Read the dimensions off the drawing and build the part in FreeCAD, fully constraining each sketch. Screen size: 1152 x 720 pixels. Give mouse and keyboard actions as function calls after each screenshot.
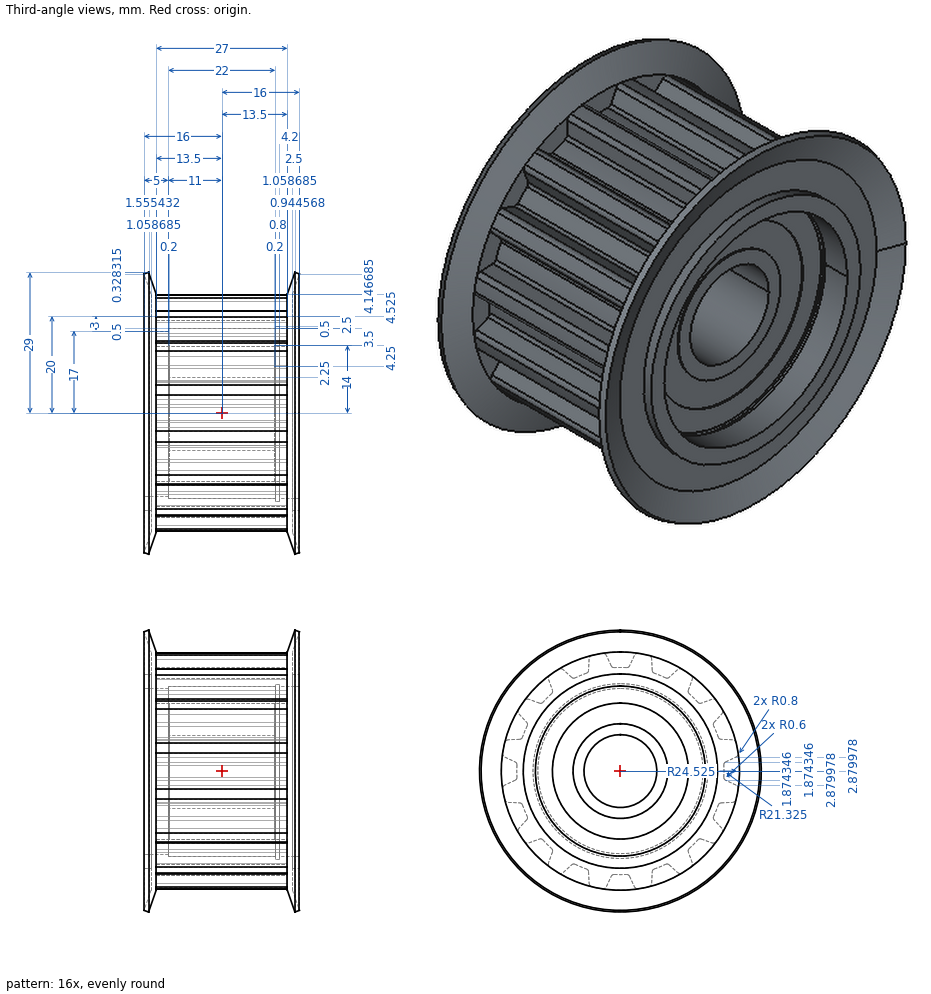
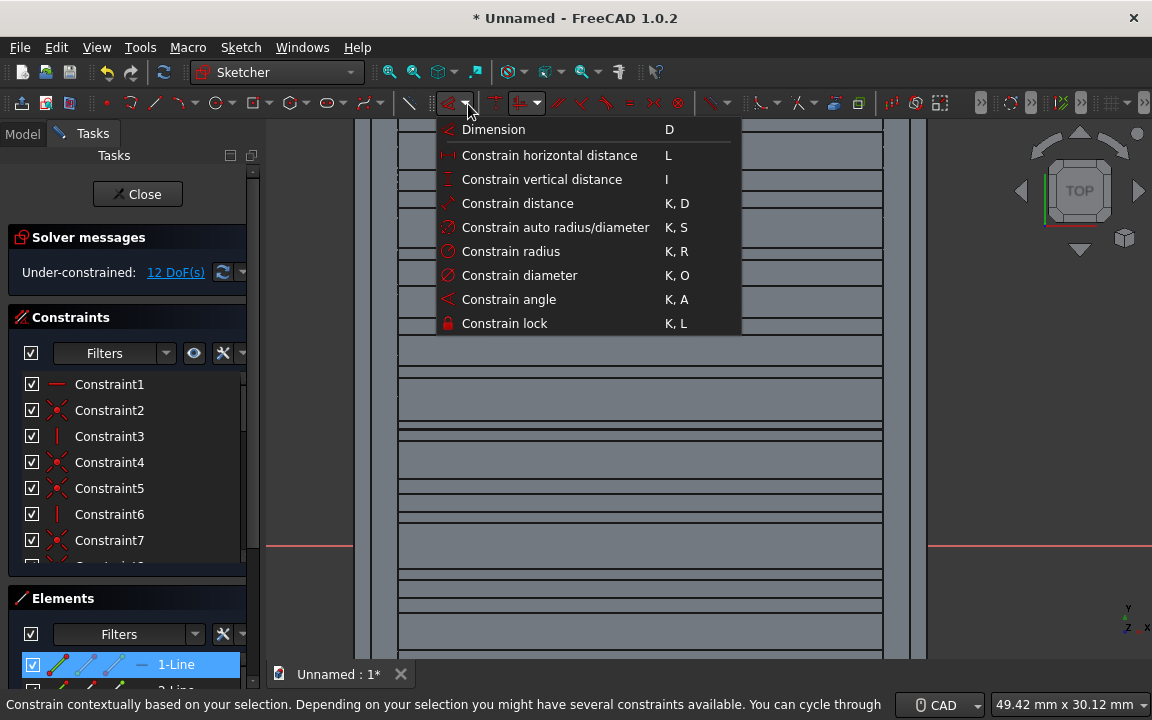
click(589, 155)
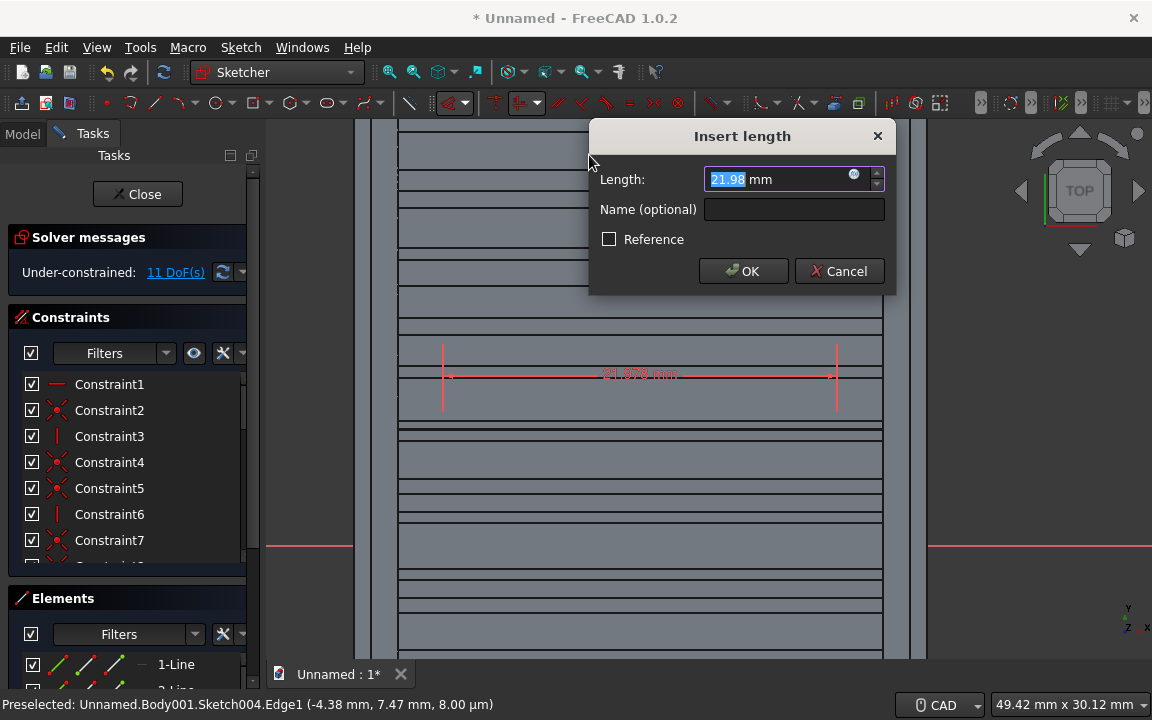
text(22)
key(Return)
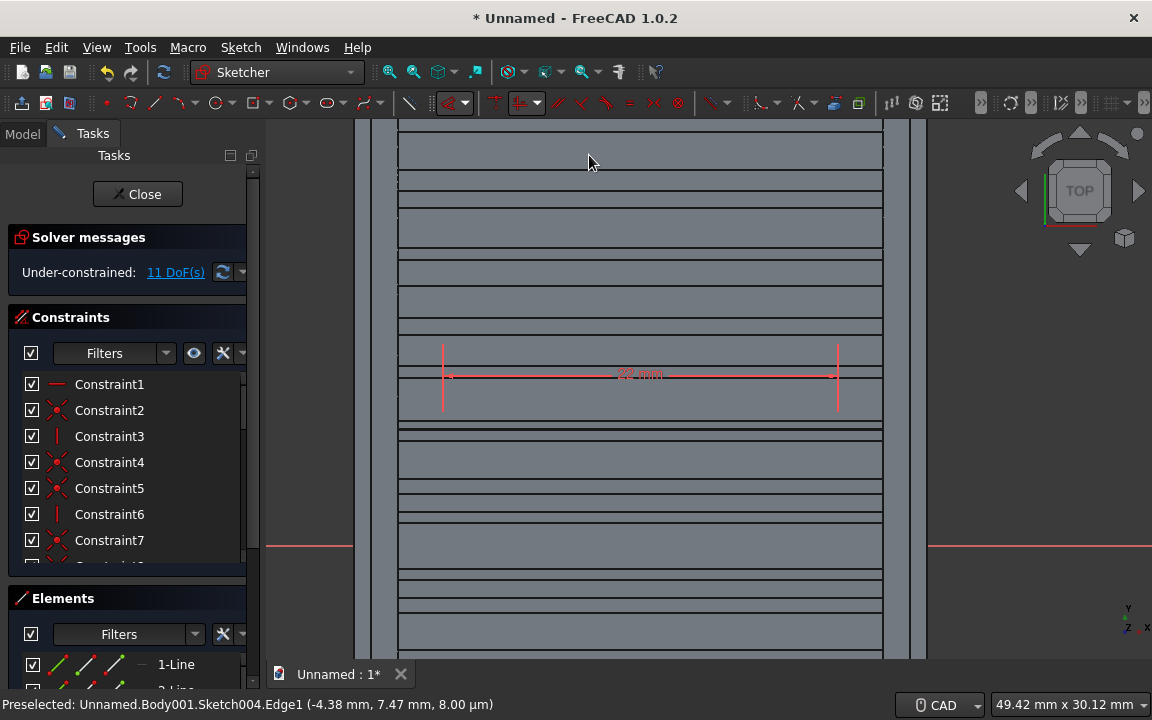
click(719, 233)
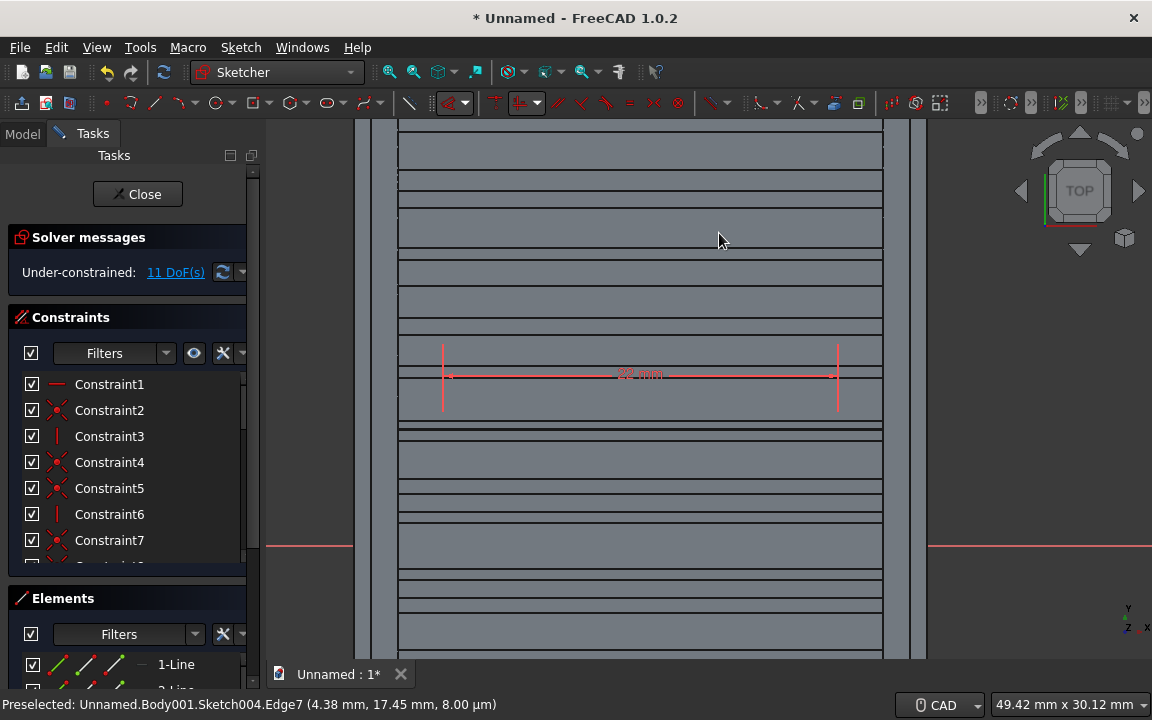
click(468, 104)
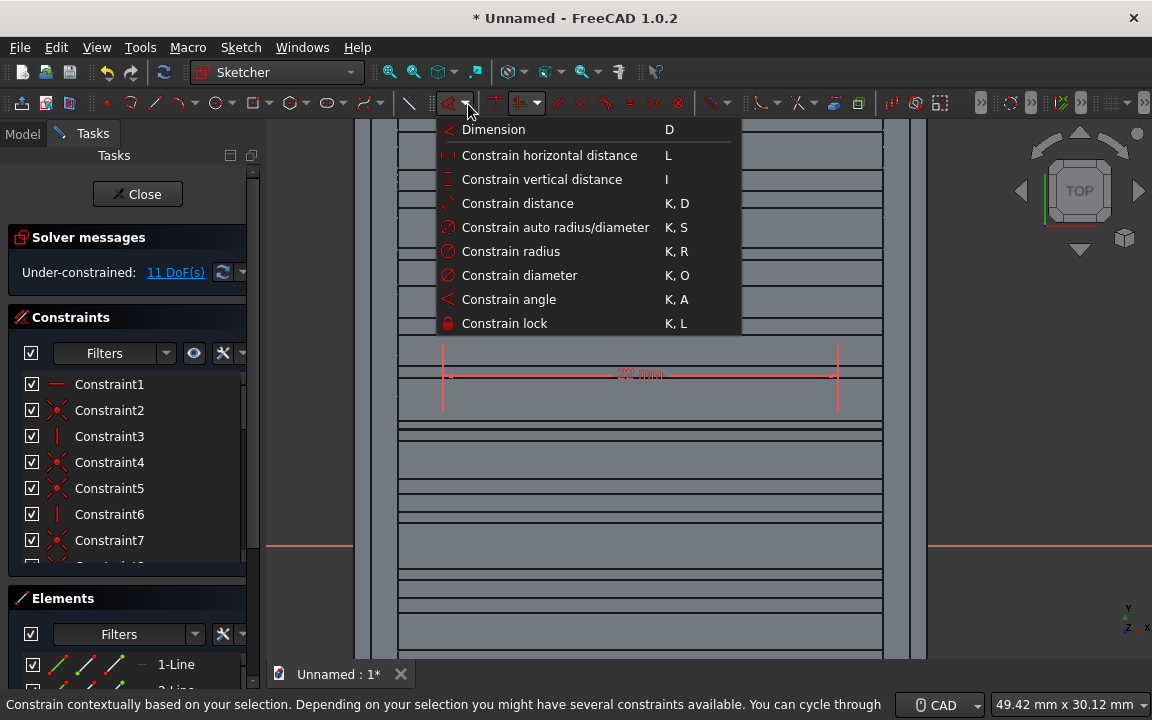
click(589, 155)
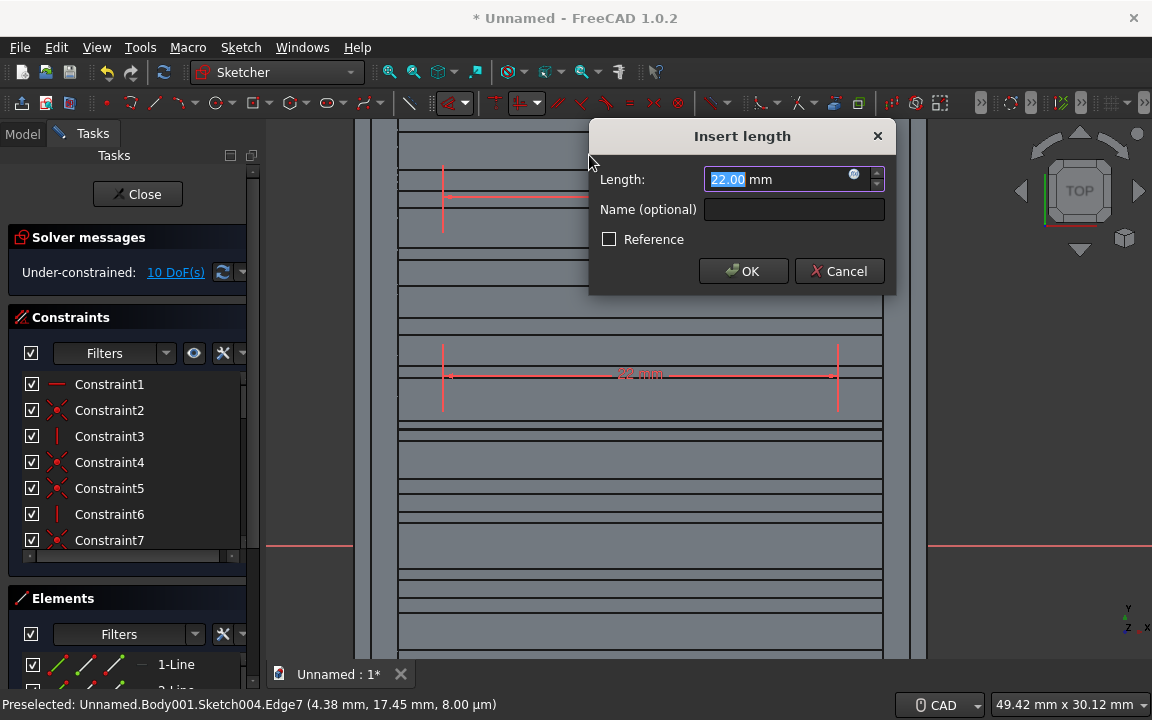
text(22)
key(Return)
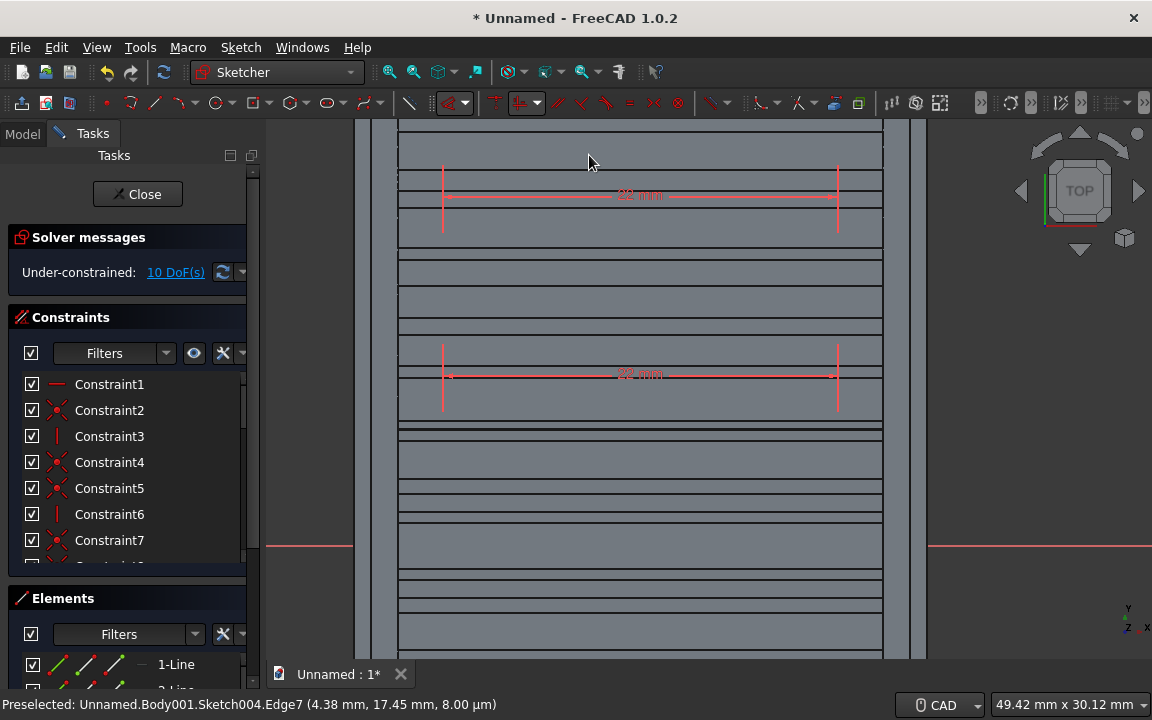
scroll(836, 372, up, 13)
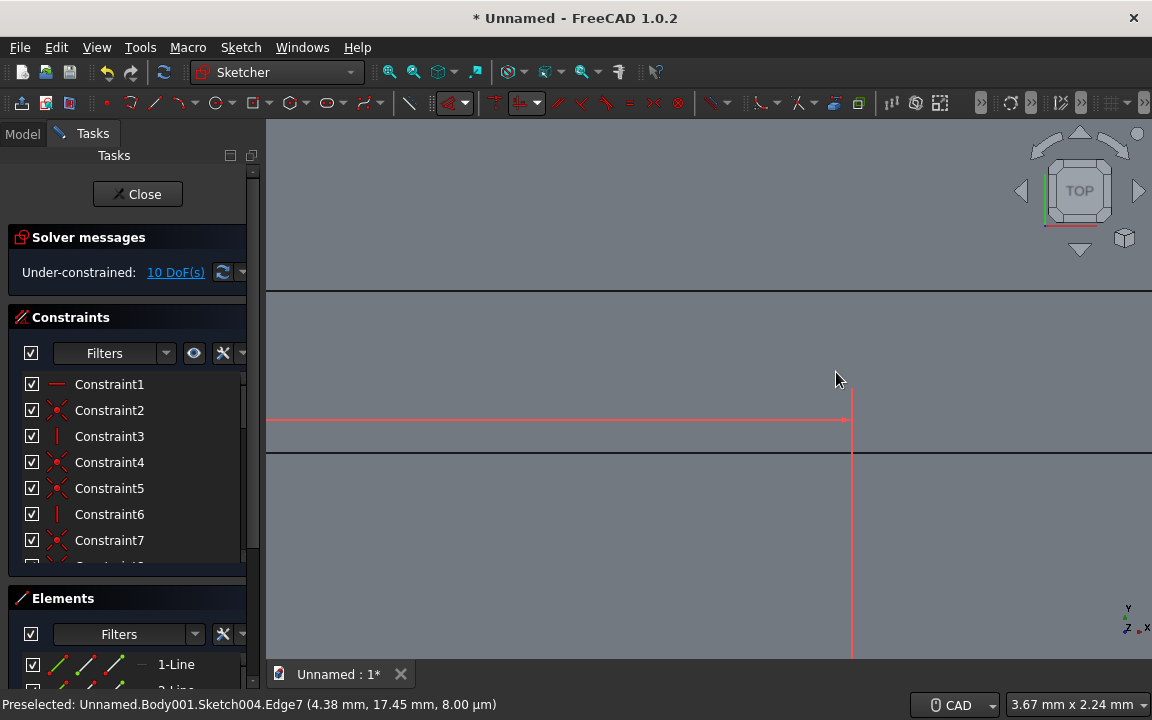
click(827, 366)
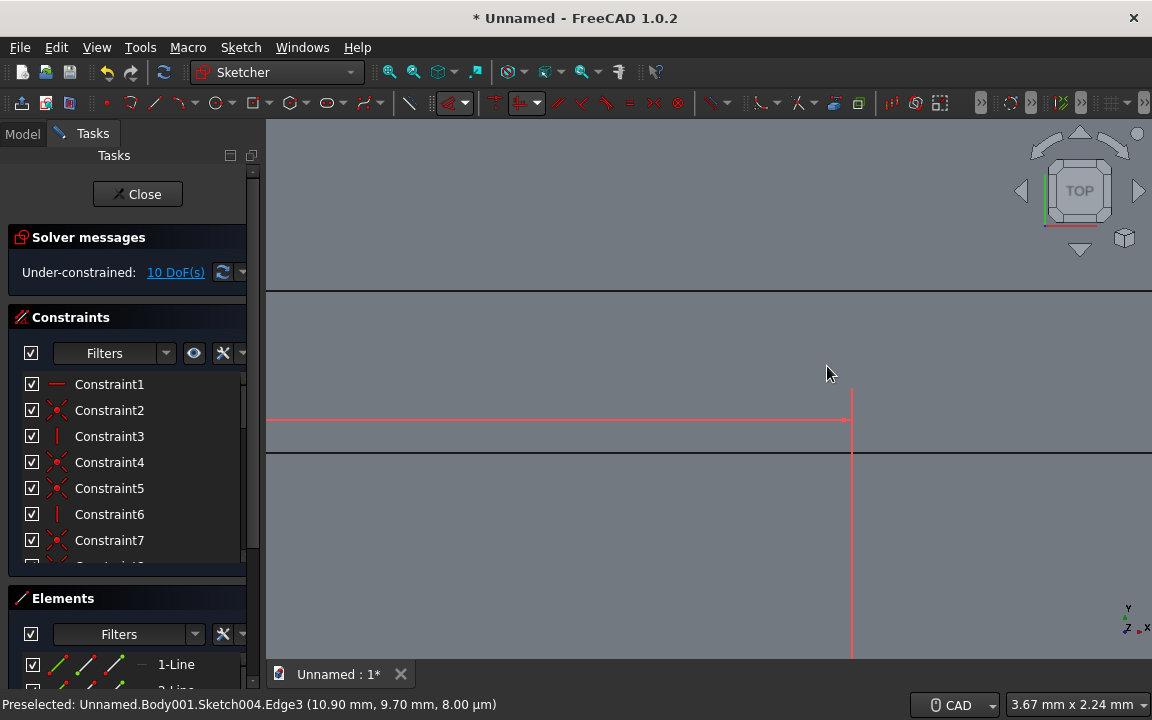
click(468, 104)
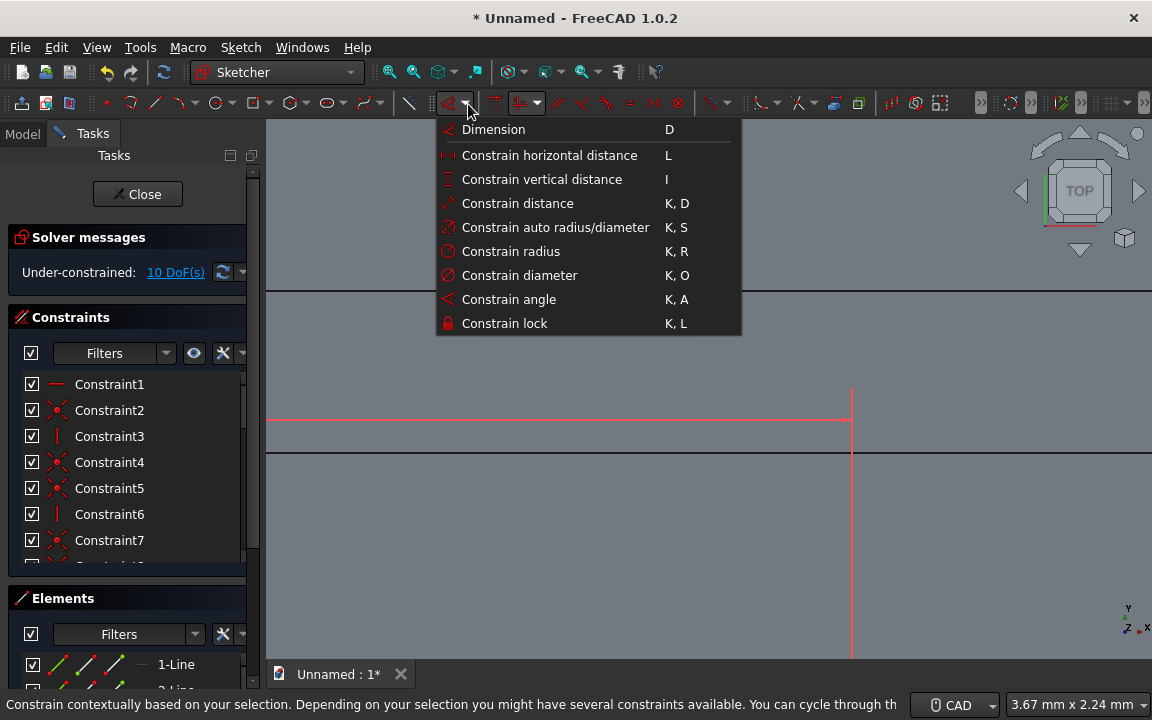
click(589, 155)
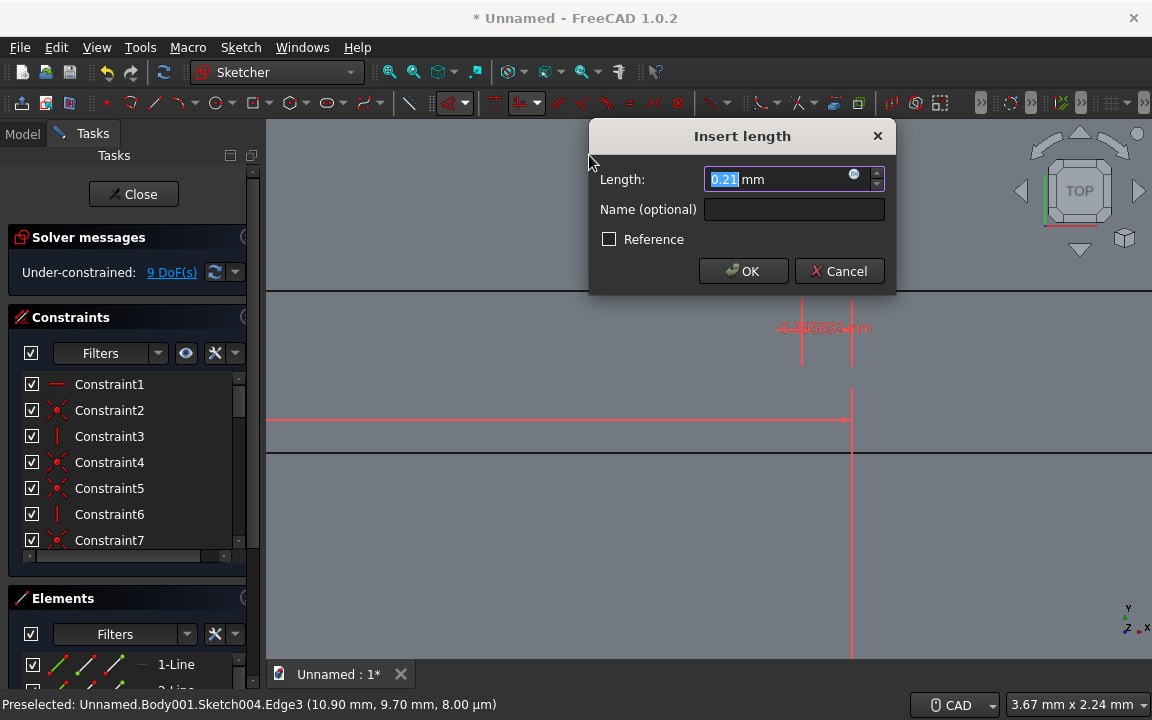
text(0.2)
key(Return)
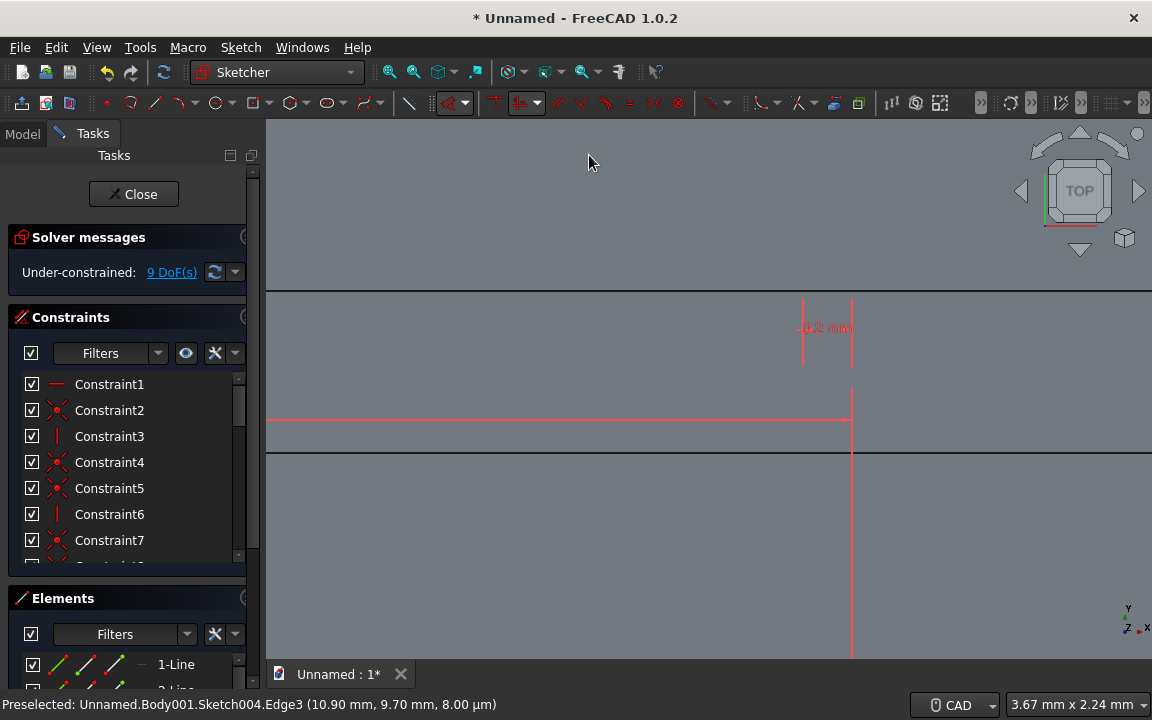
scroll(837, 372, down, 13)